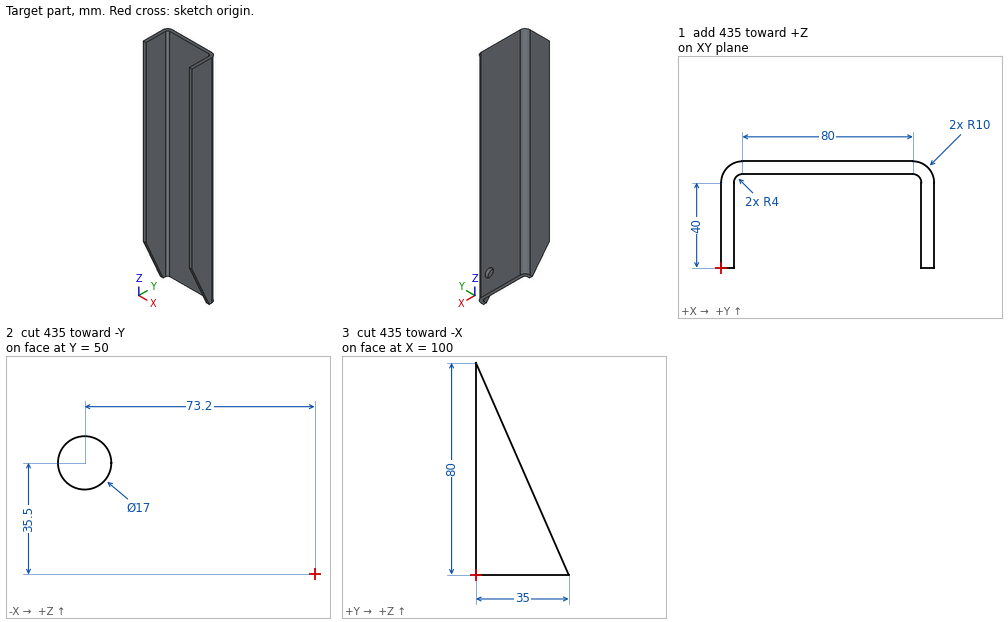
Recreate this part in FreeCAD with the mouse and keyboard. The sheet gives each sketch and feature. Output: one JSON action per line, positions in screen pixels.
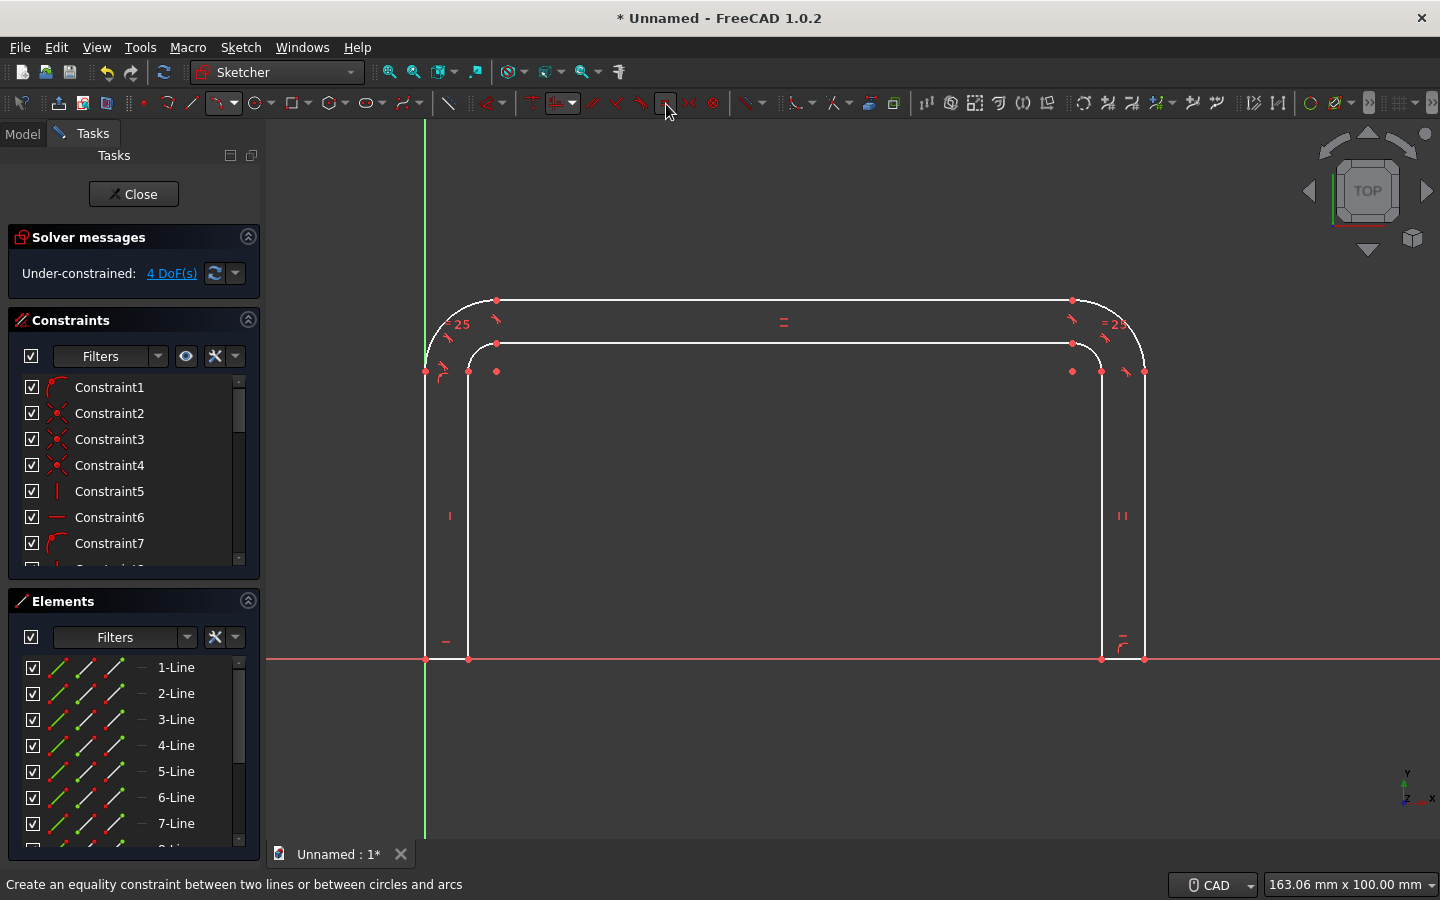
{"action": "scroll", "coordinate": [484, 346], "scroll_direction": "up", "scroll_amount": 2}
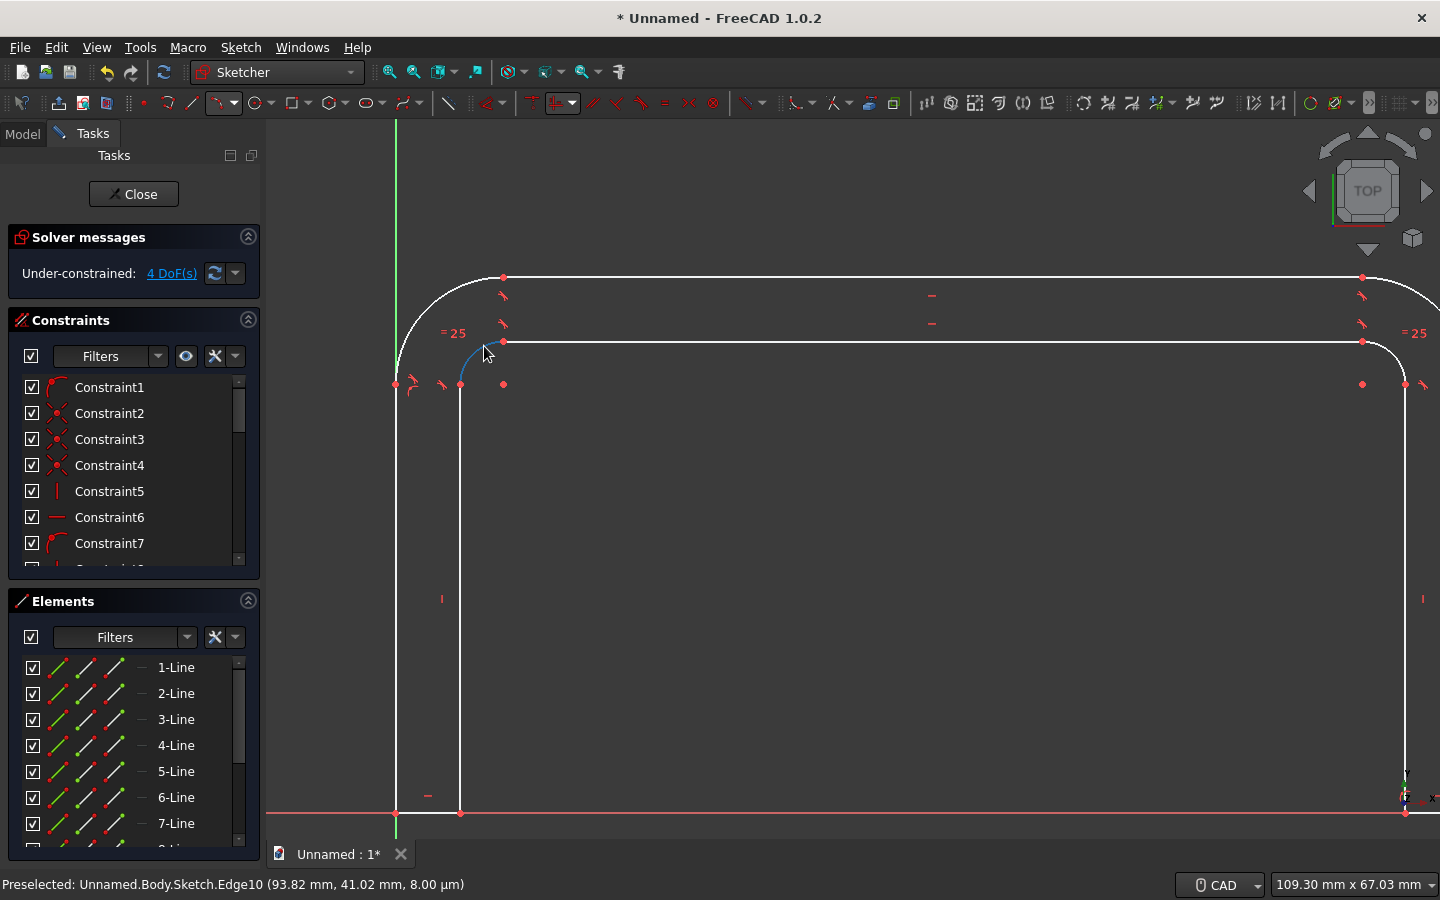
{"action": "left_click", "coordinate": [484, 346]}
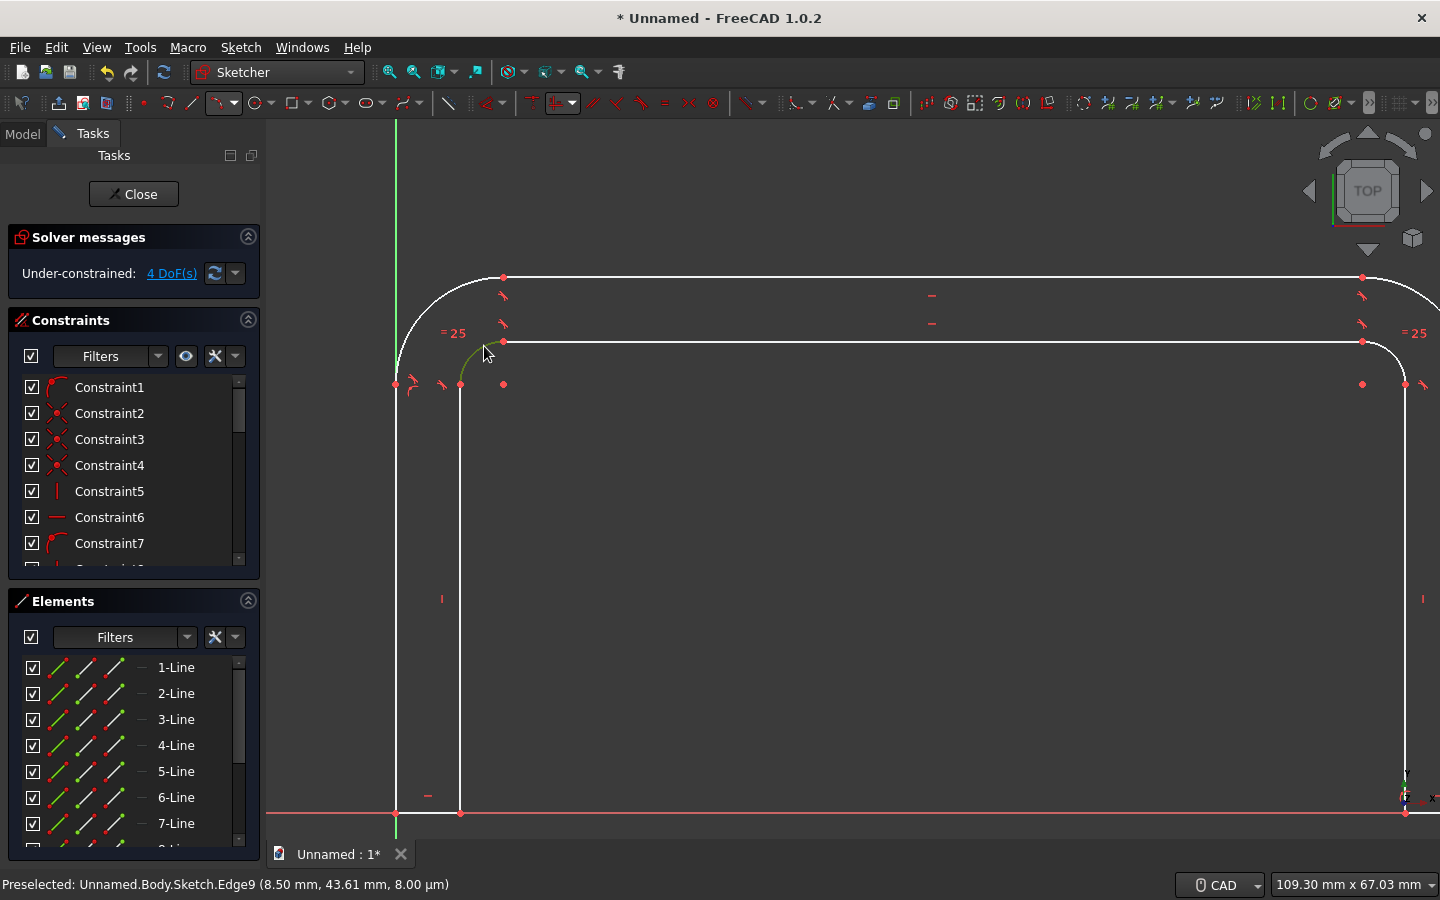
{"action": "left_click", "coordinate": [504, 104]}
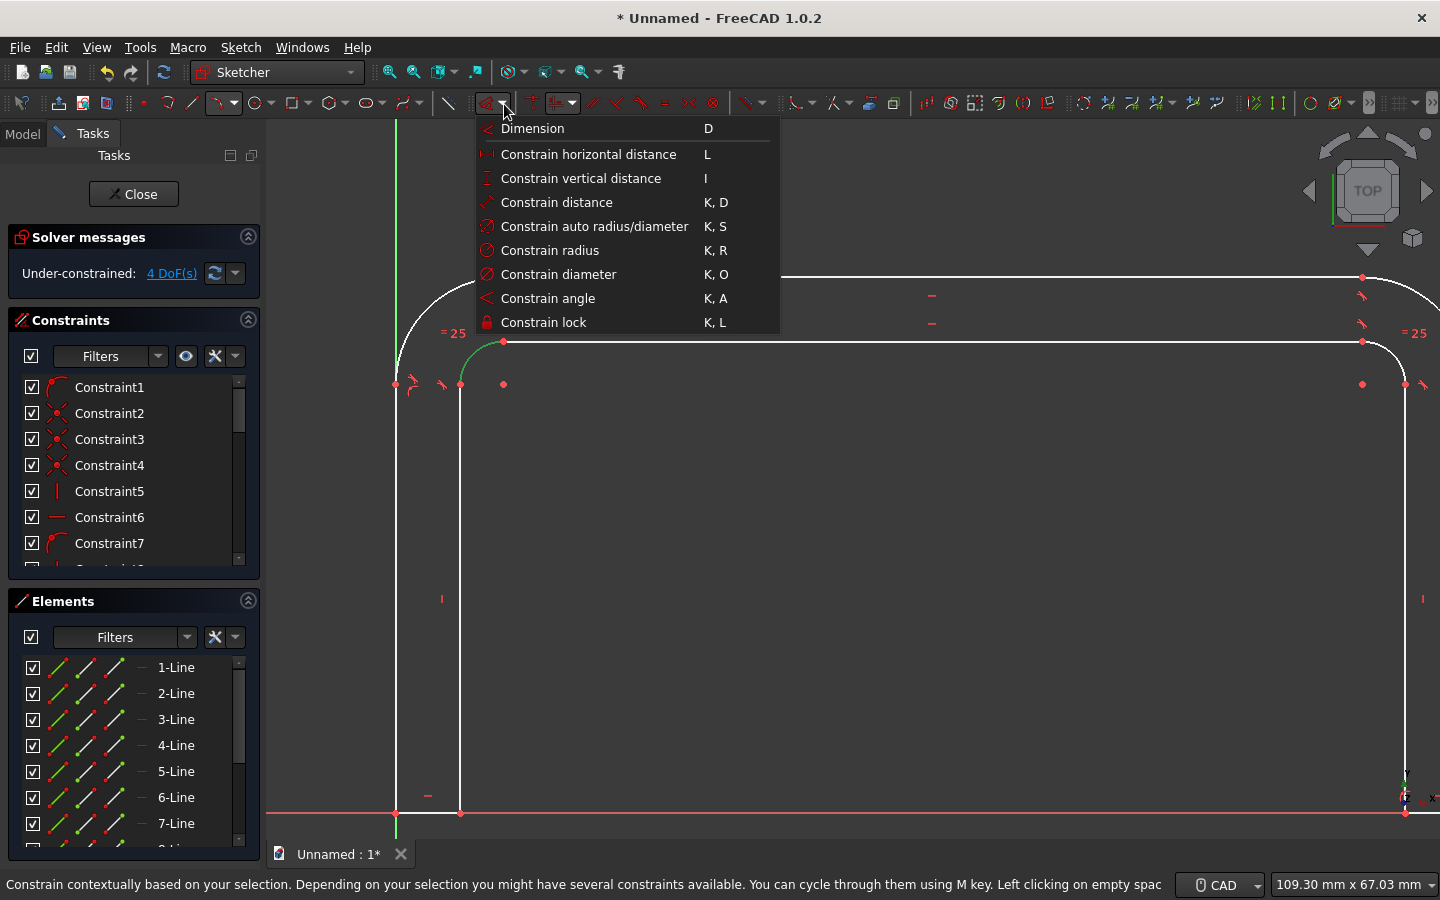
{"action": "left_click", "coordinate": [628, 250]}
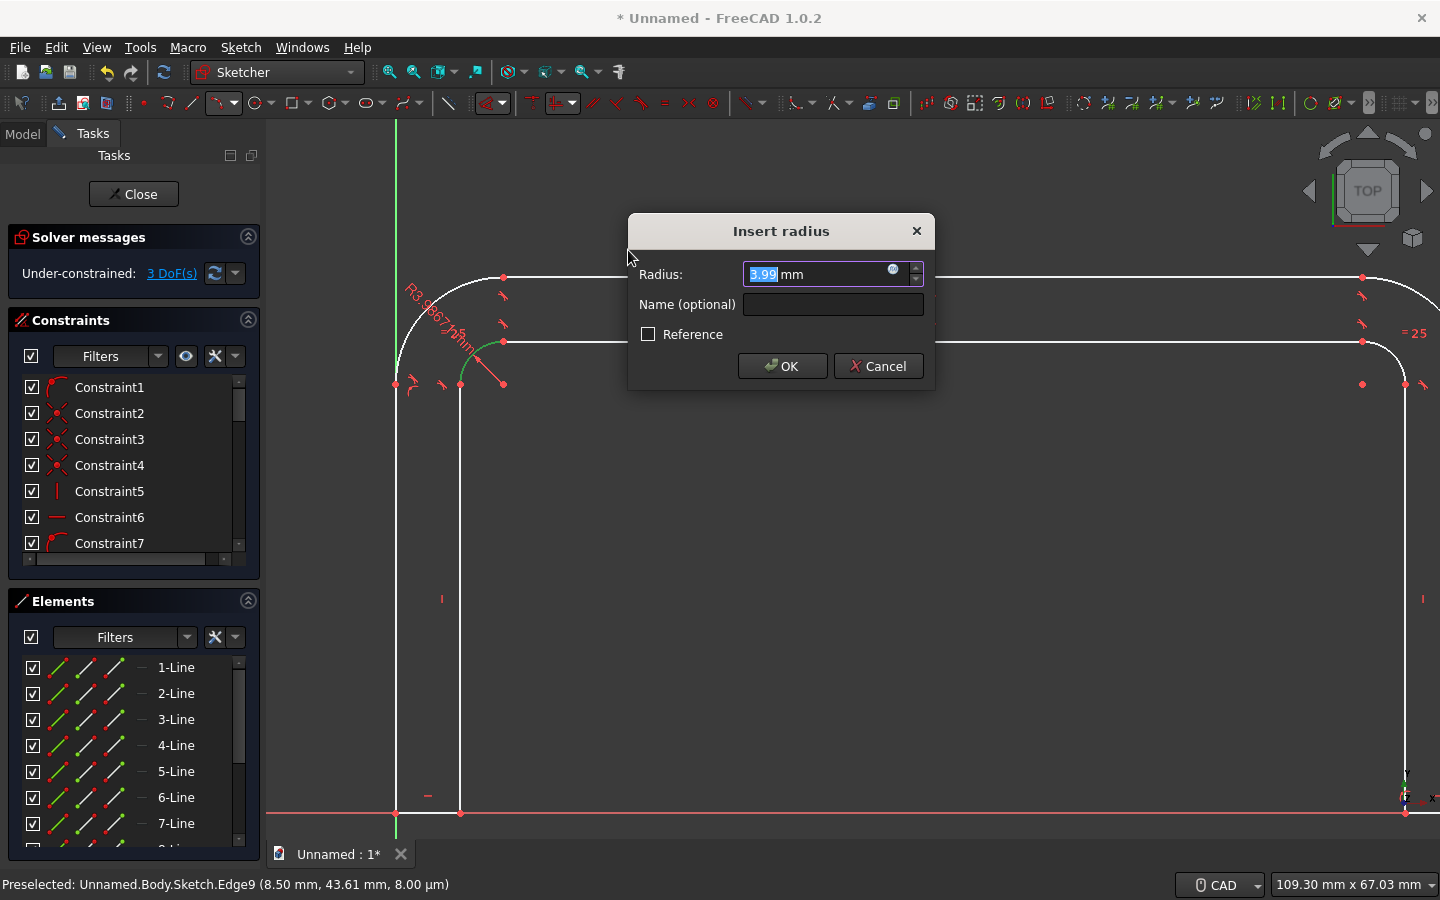
{"action": "type", "text": "4"}
{"action": "key", "text": "Return"}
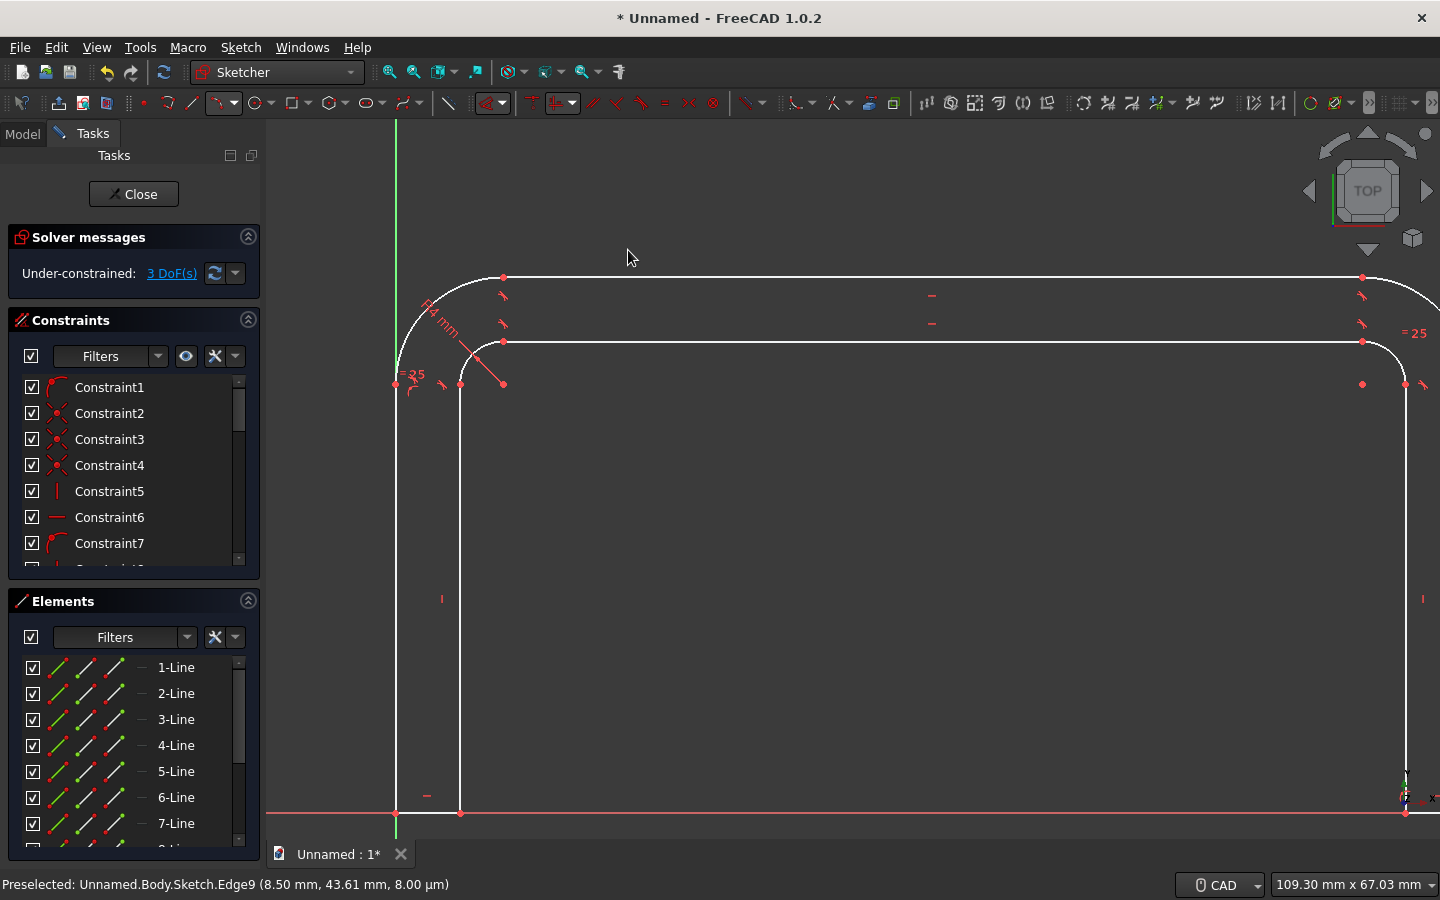
{"action": "scroll", "coordinate": [483, 345], "scroll_direction": "down", "scroll_amount": 2}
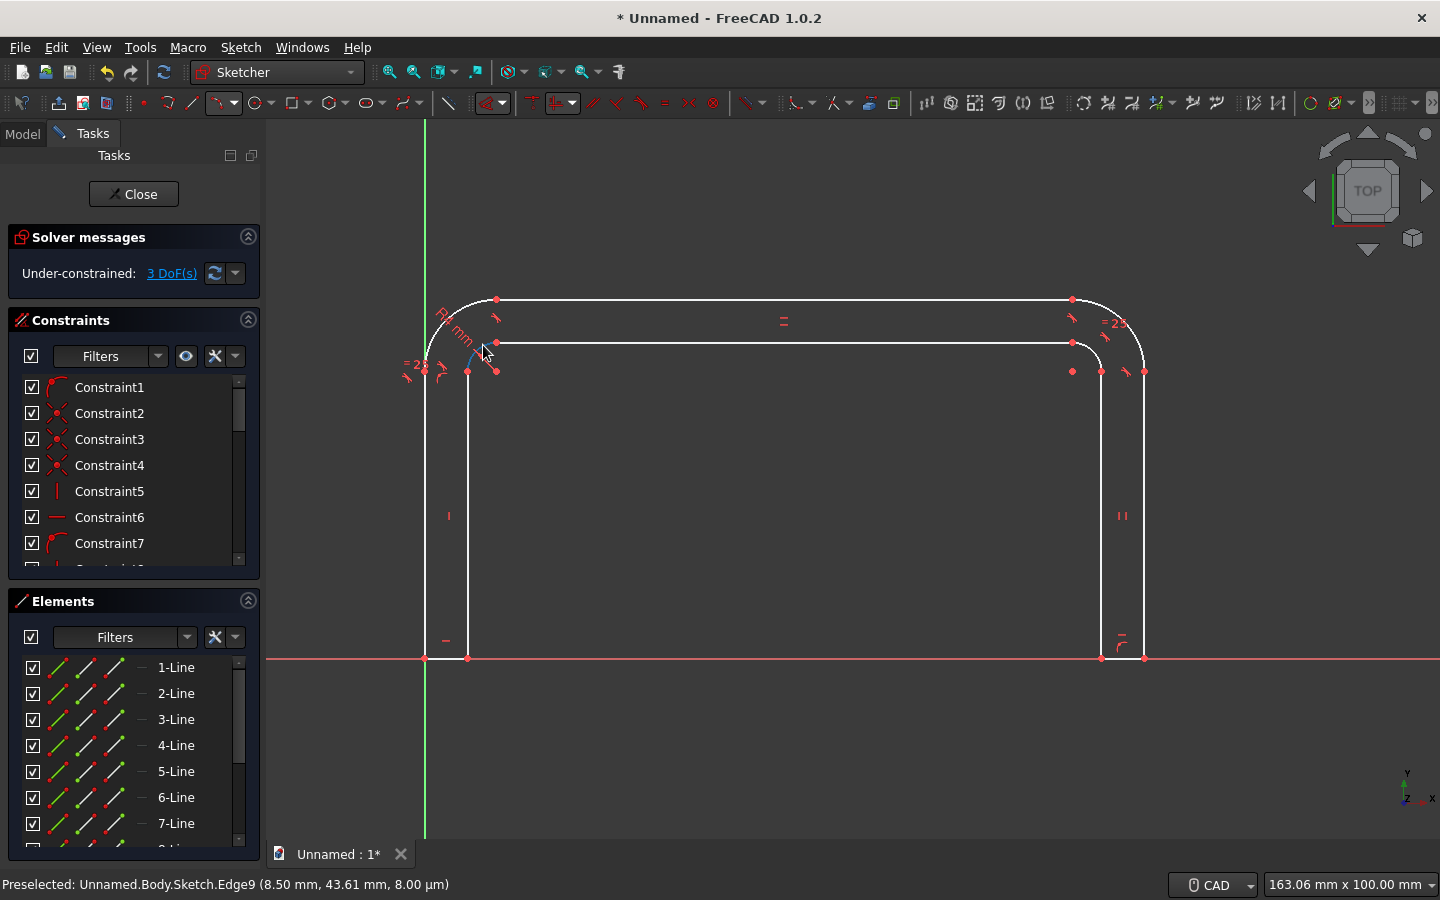
{"action": "left_click", "coordinate": [1137, 339]}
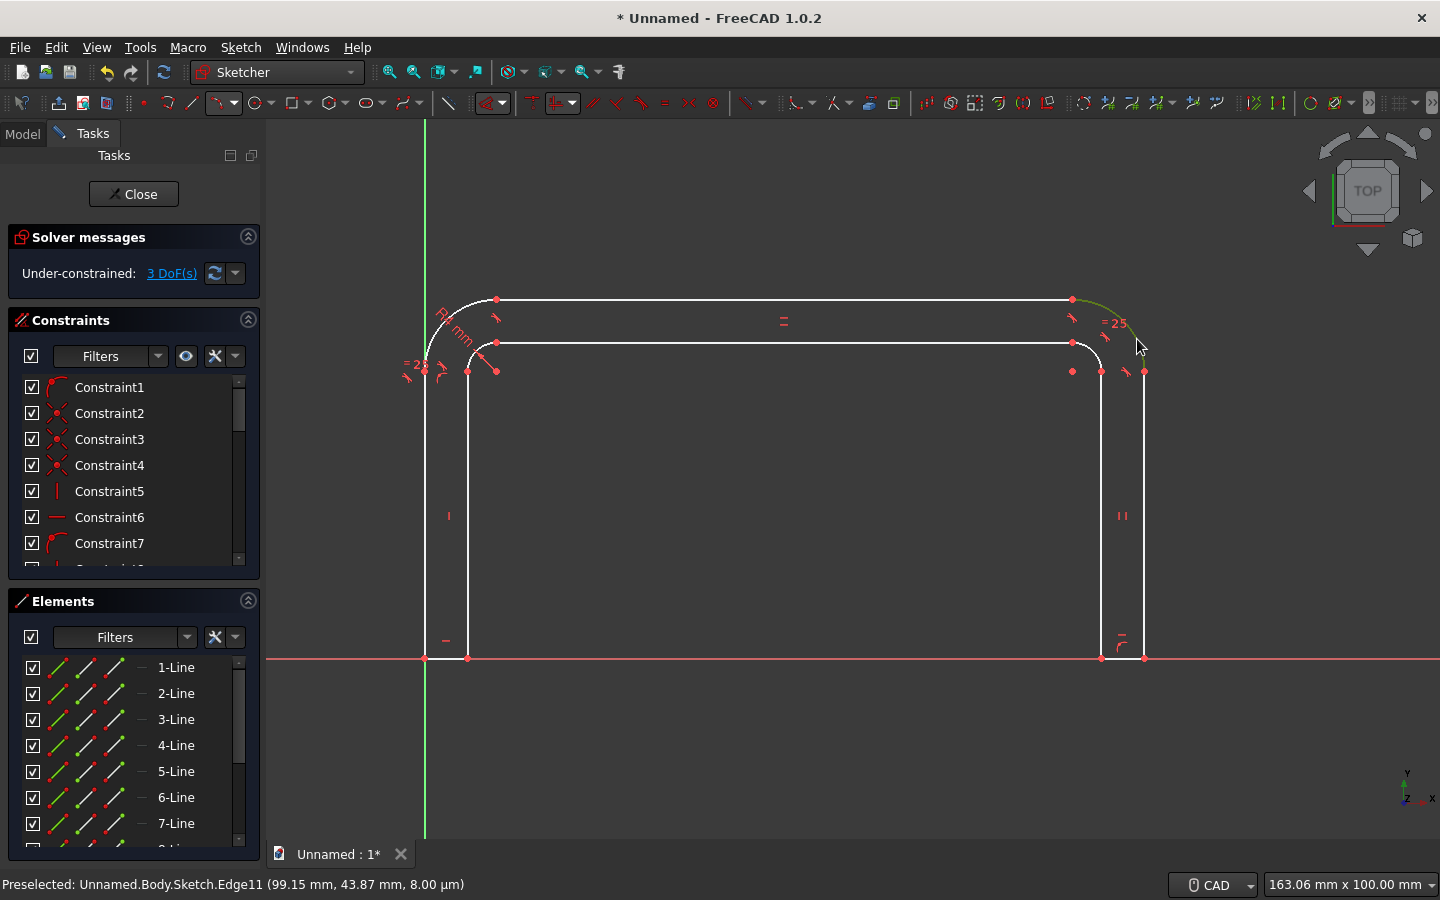
{"action": "key", "text": "k r"}